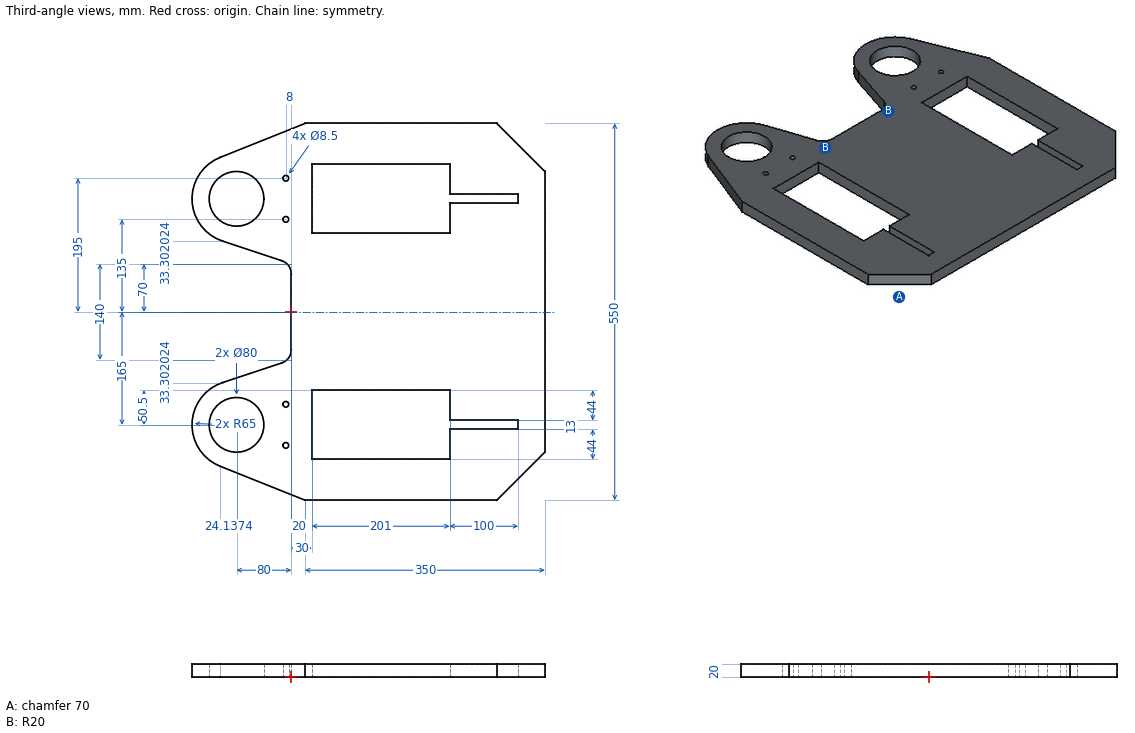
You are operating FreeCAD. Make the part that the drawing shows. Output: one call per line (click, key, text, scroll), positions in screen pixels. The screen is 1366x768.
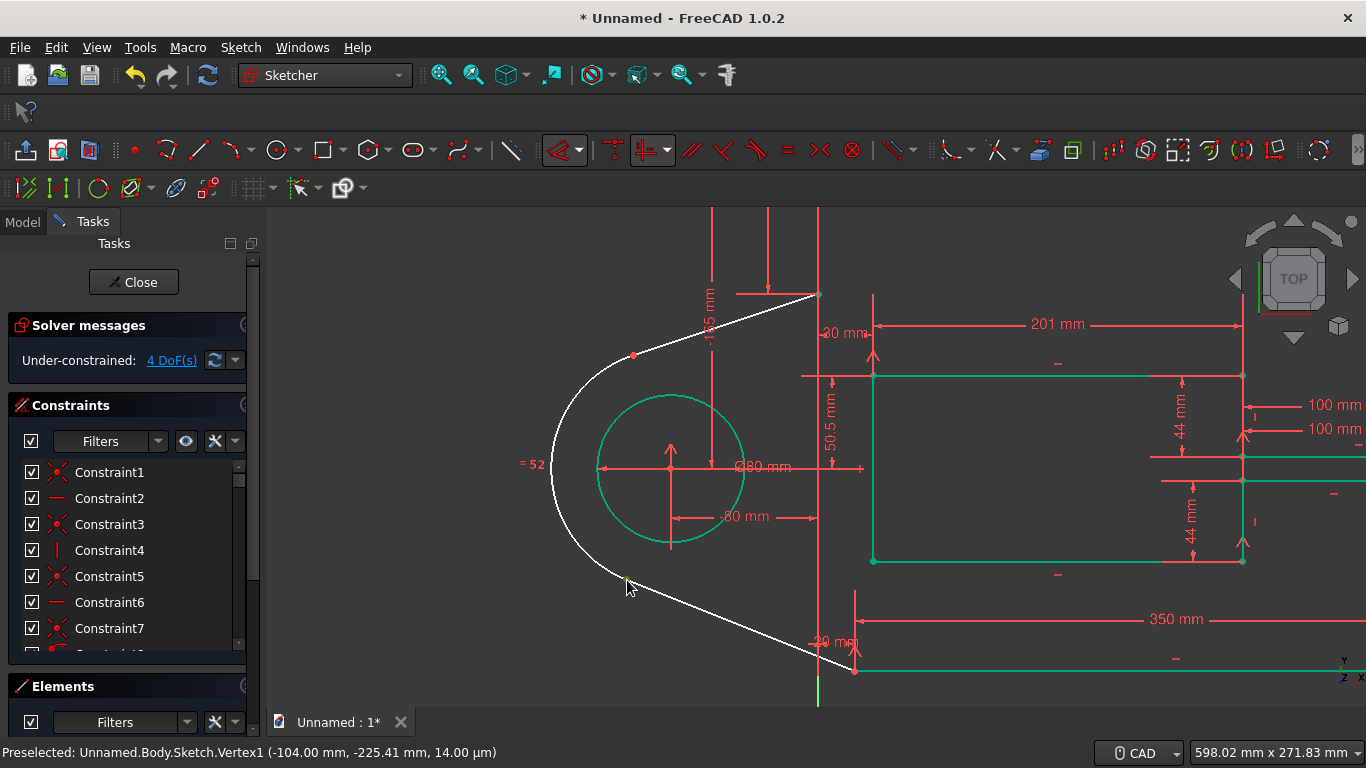
click(671, 469)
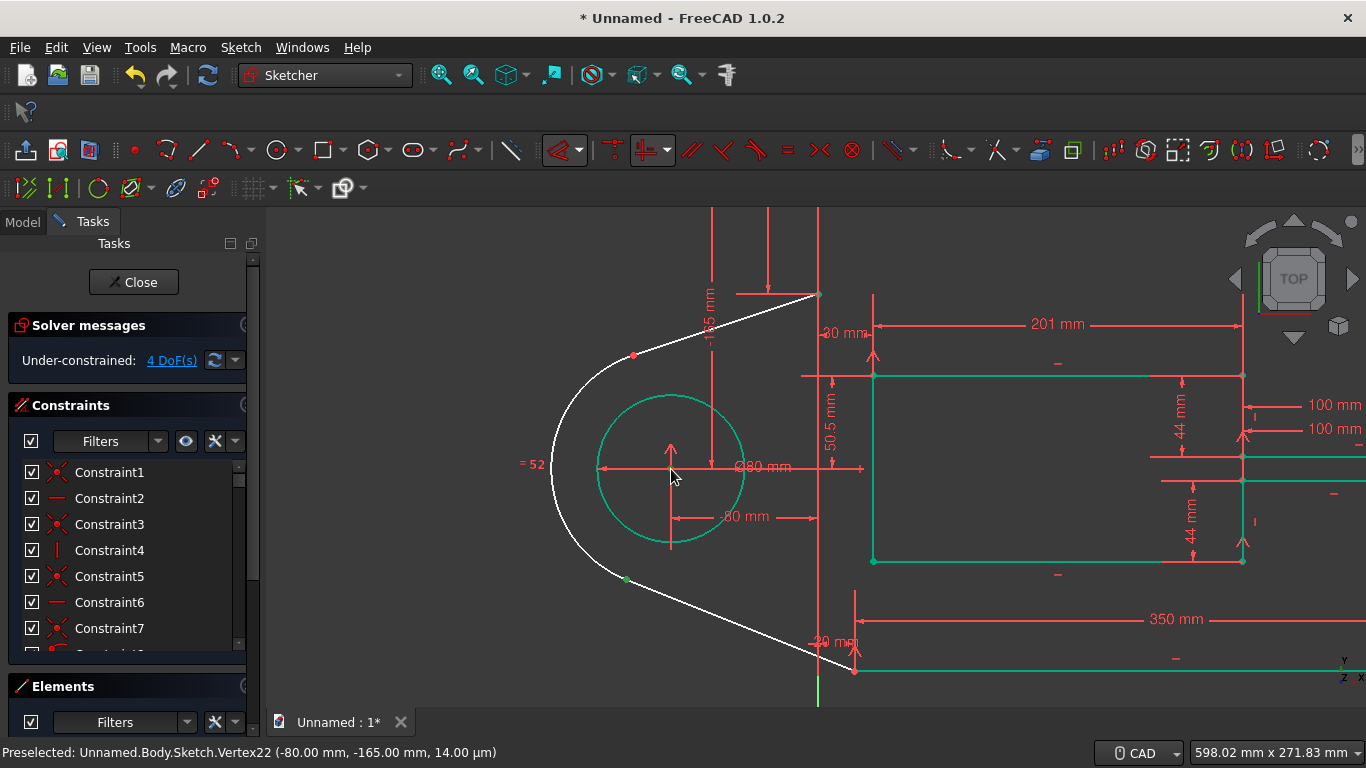
click(582, 150)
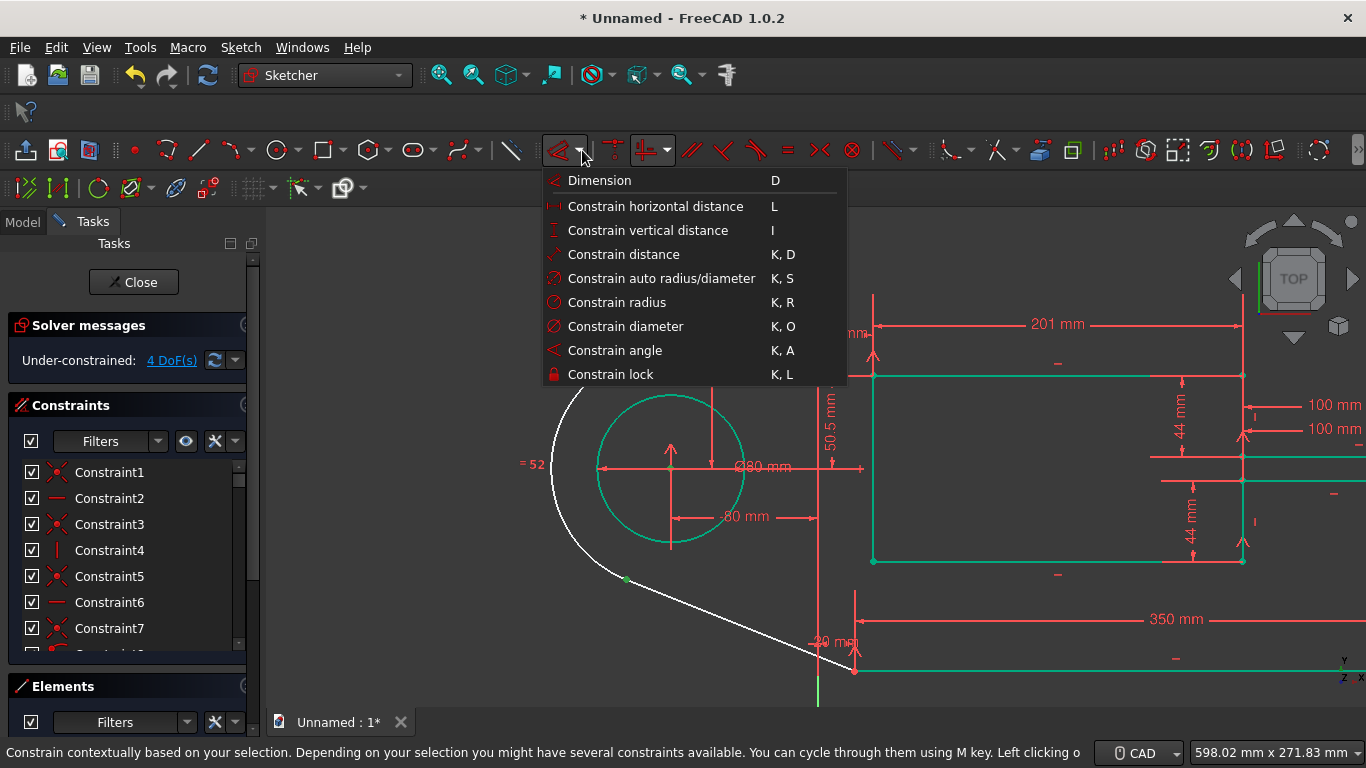
click(695, 206)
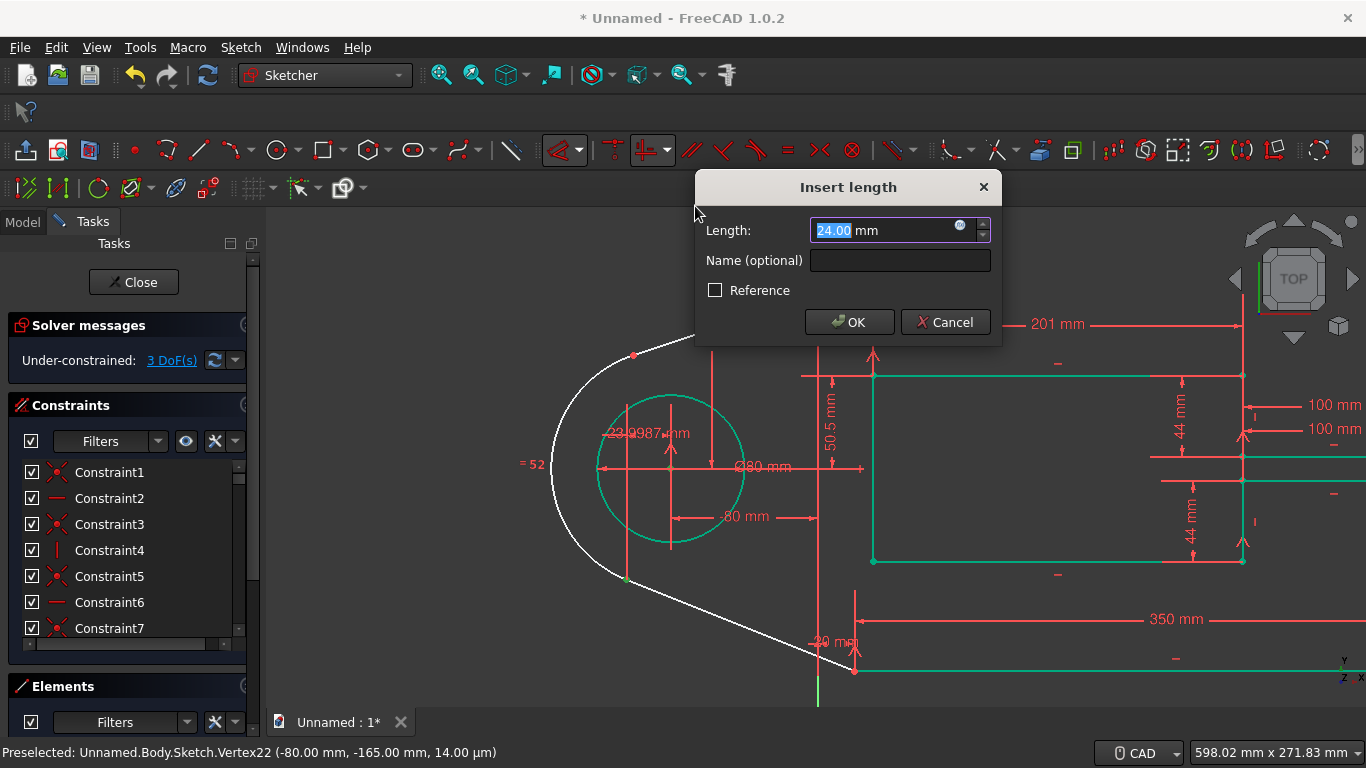
text(24.1374)
key(Return)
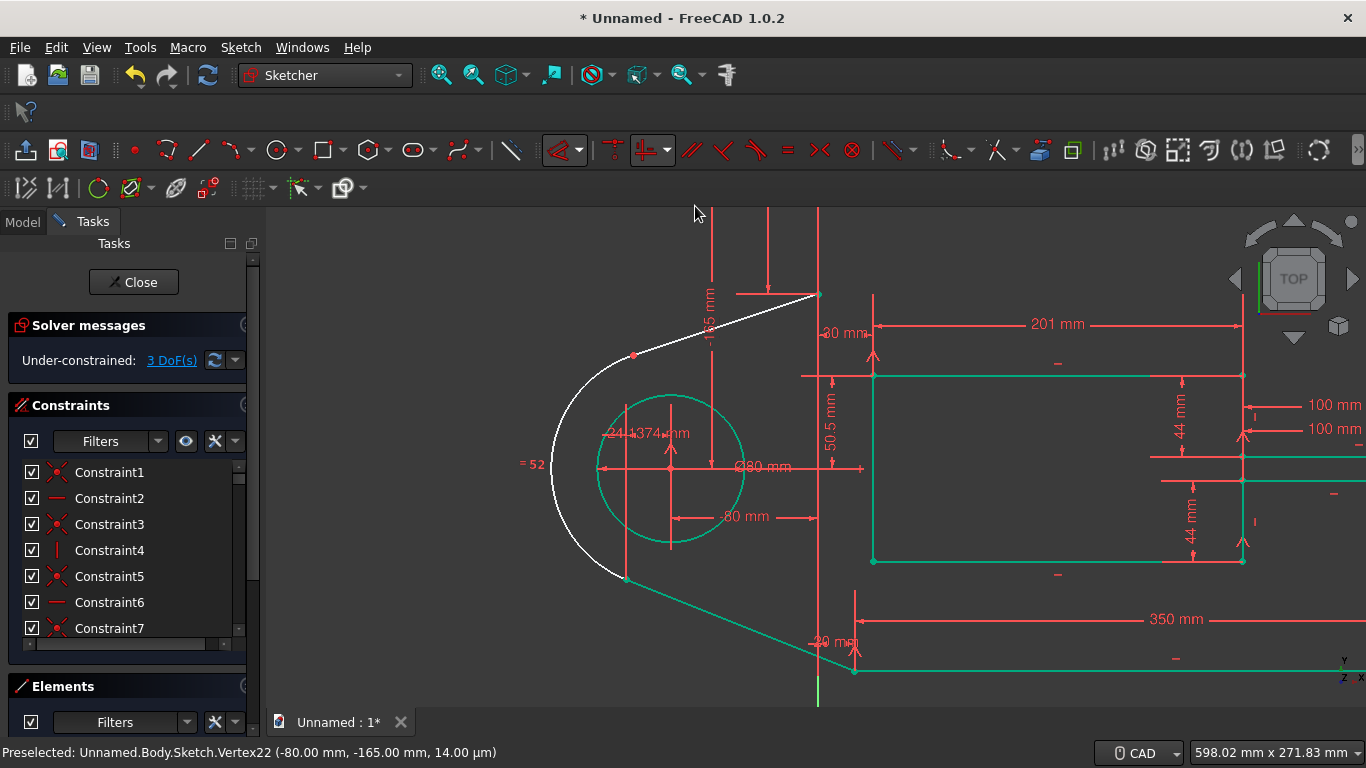
scroll(628, 583, down, 6)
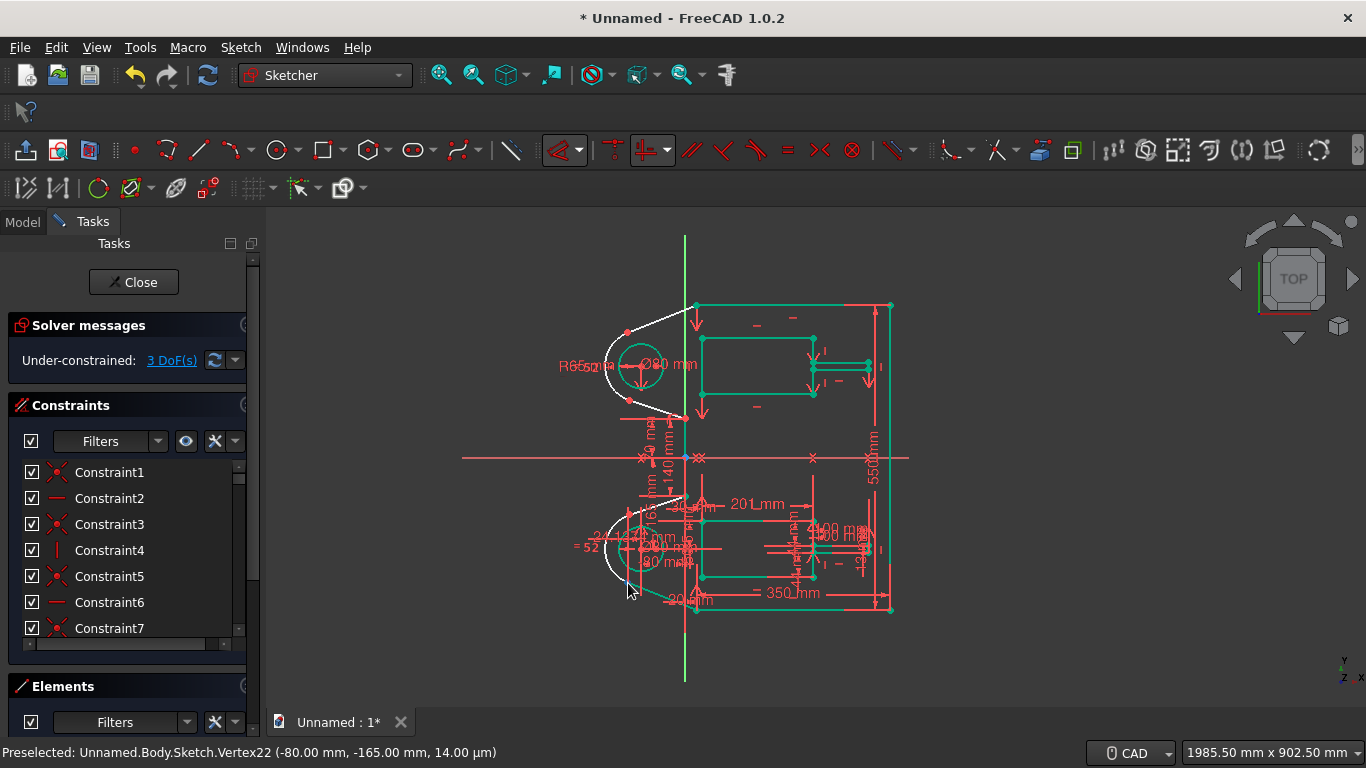
scroll(628, 333, up, 6)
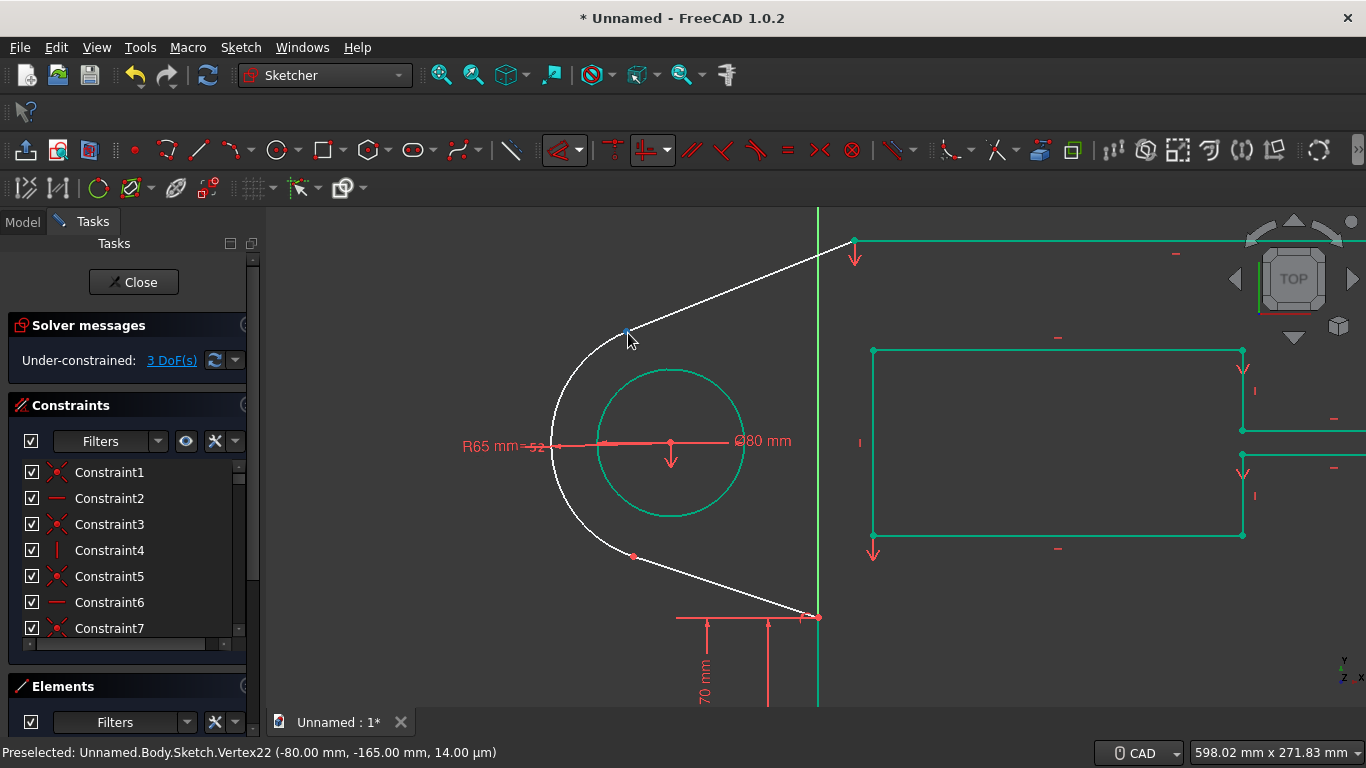
click(627, 332)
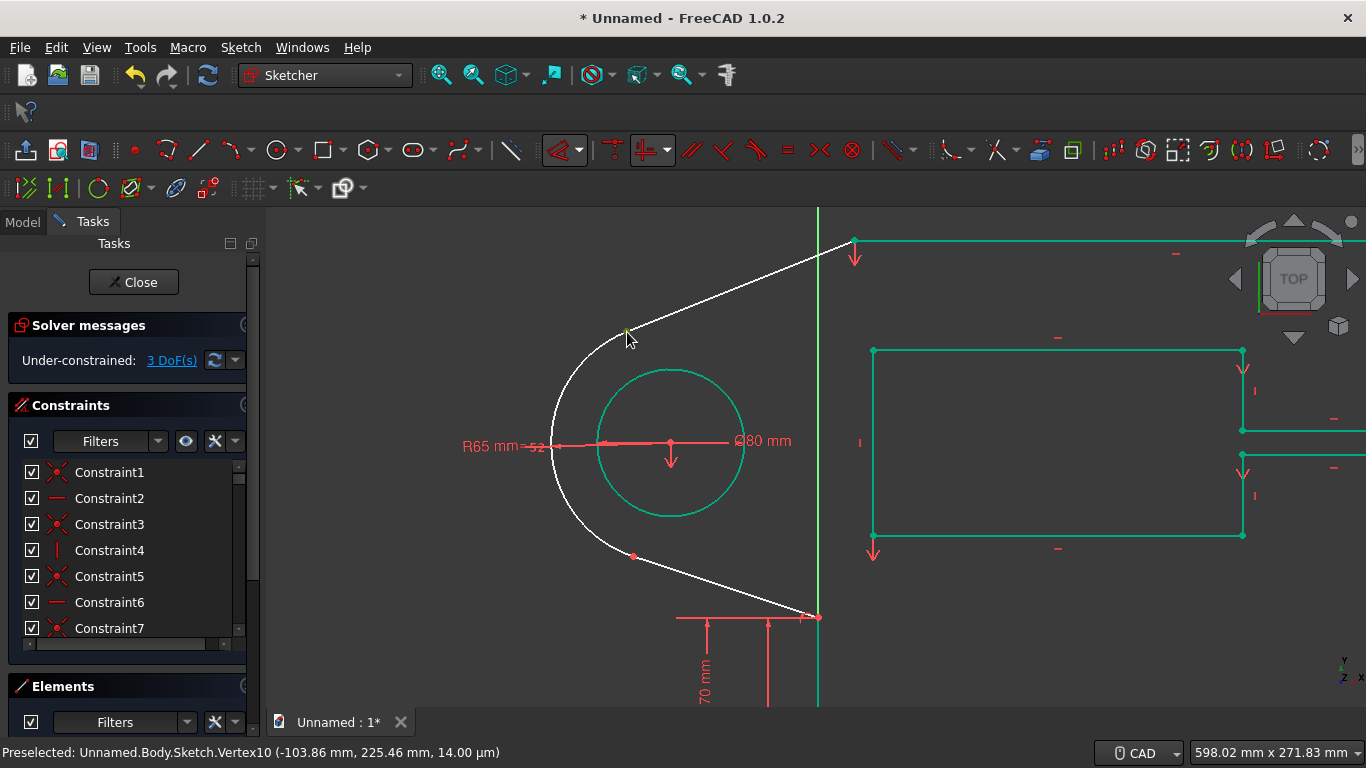
click(671, 443)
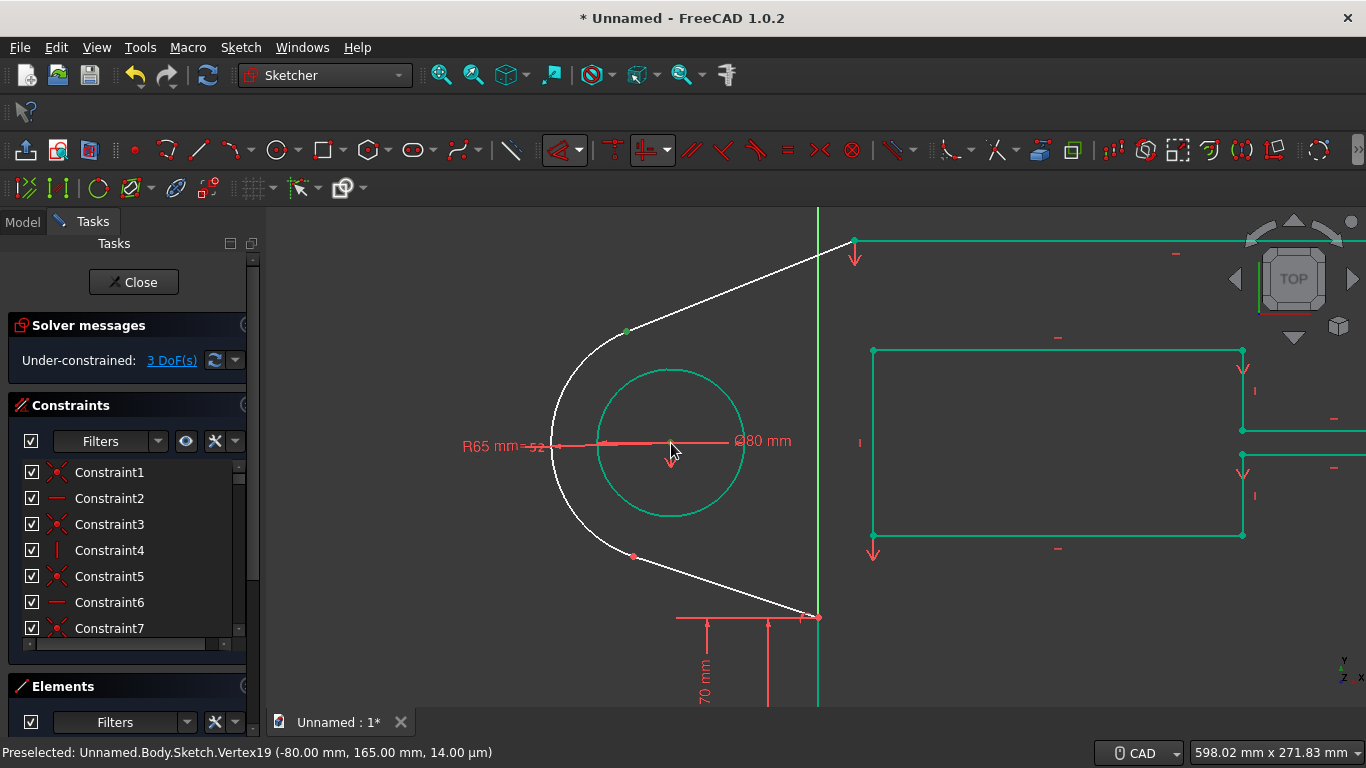
key(l)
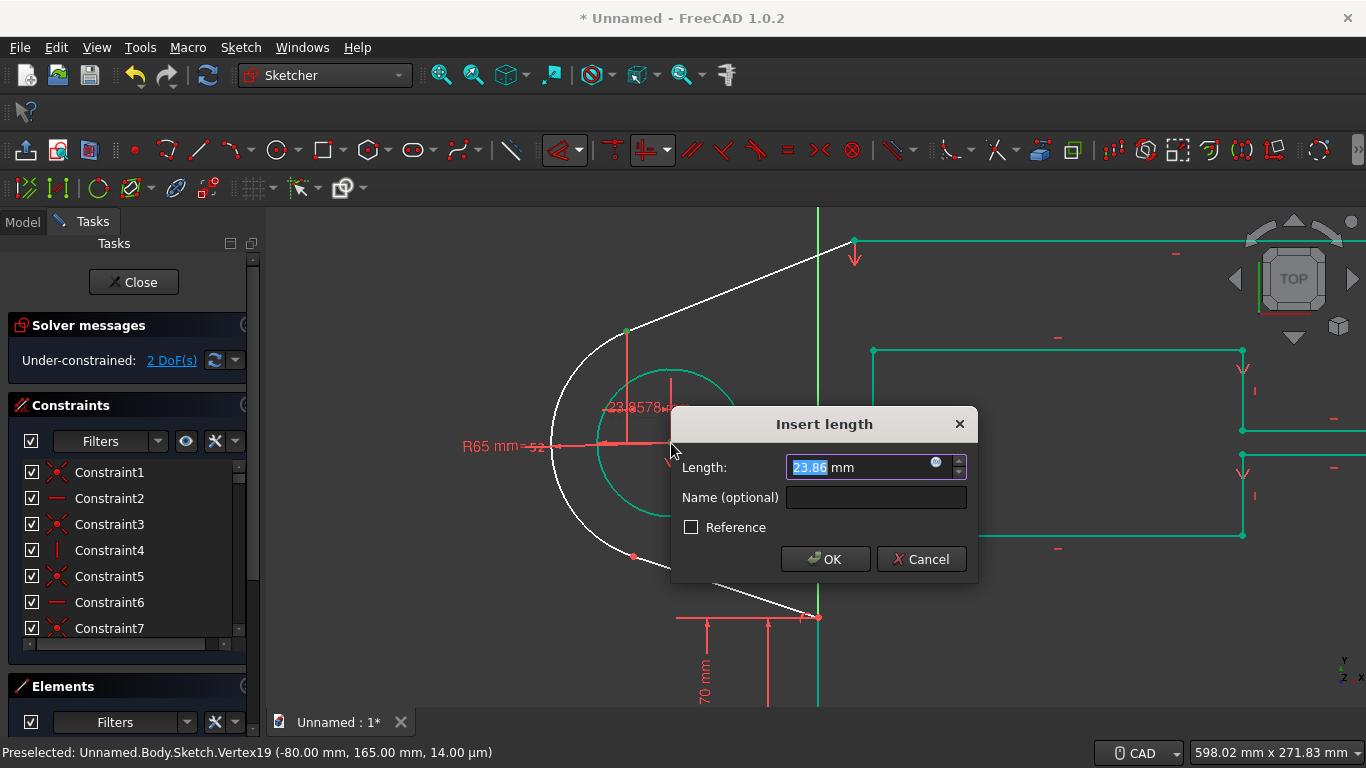
text(24.1374)
key(Return)